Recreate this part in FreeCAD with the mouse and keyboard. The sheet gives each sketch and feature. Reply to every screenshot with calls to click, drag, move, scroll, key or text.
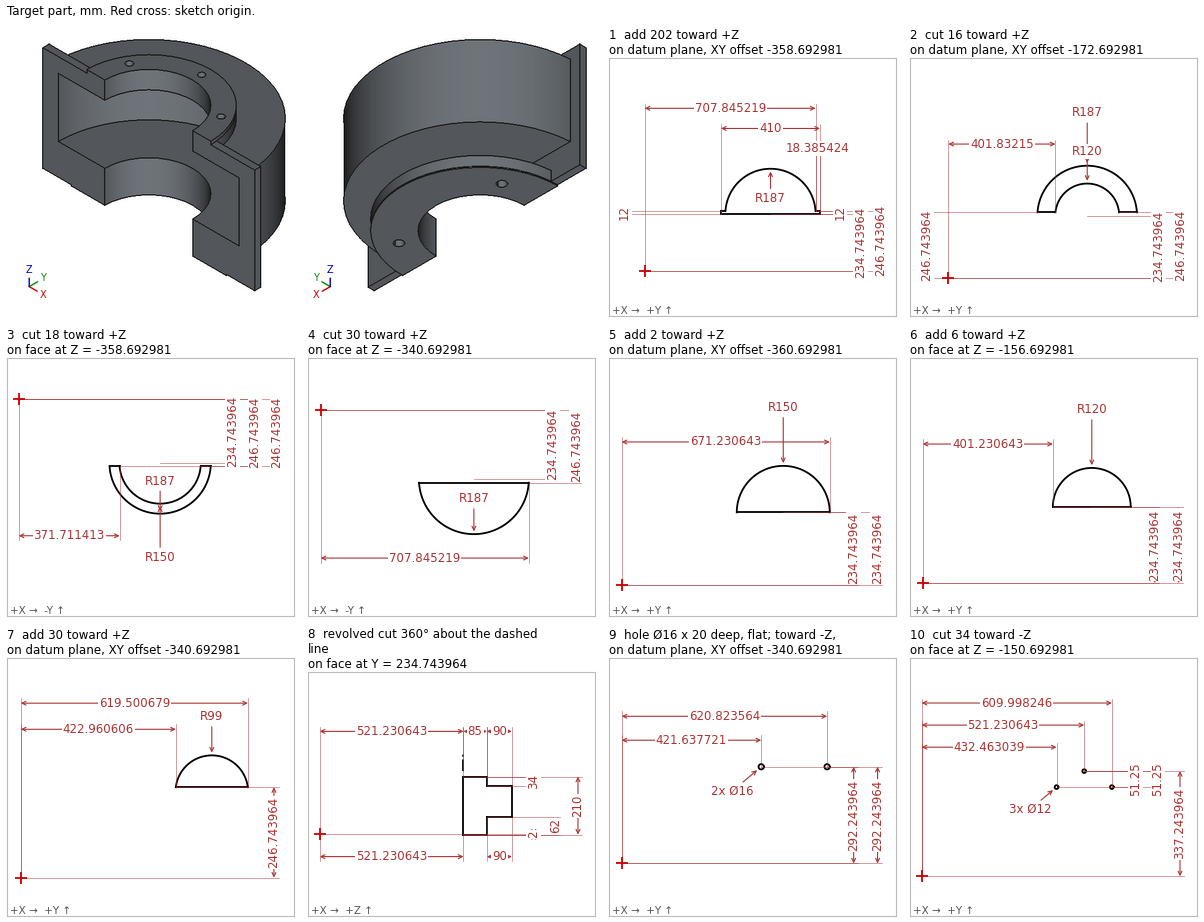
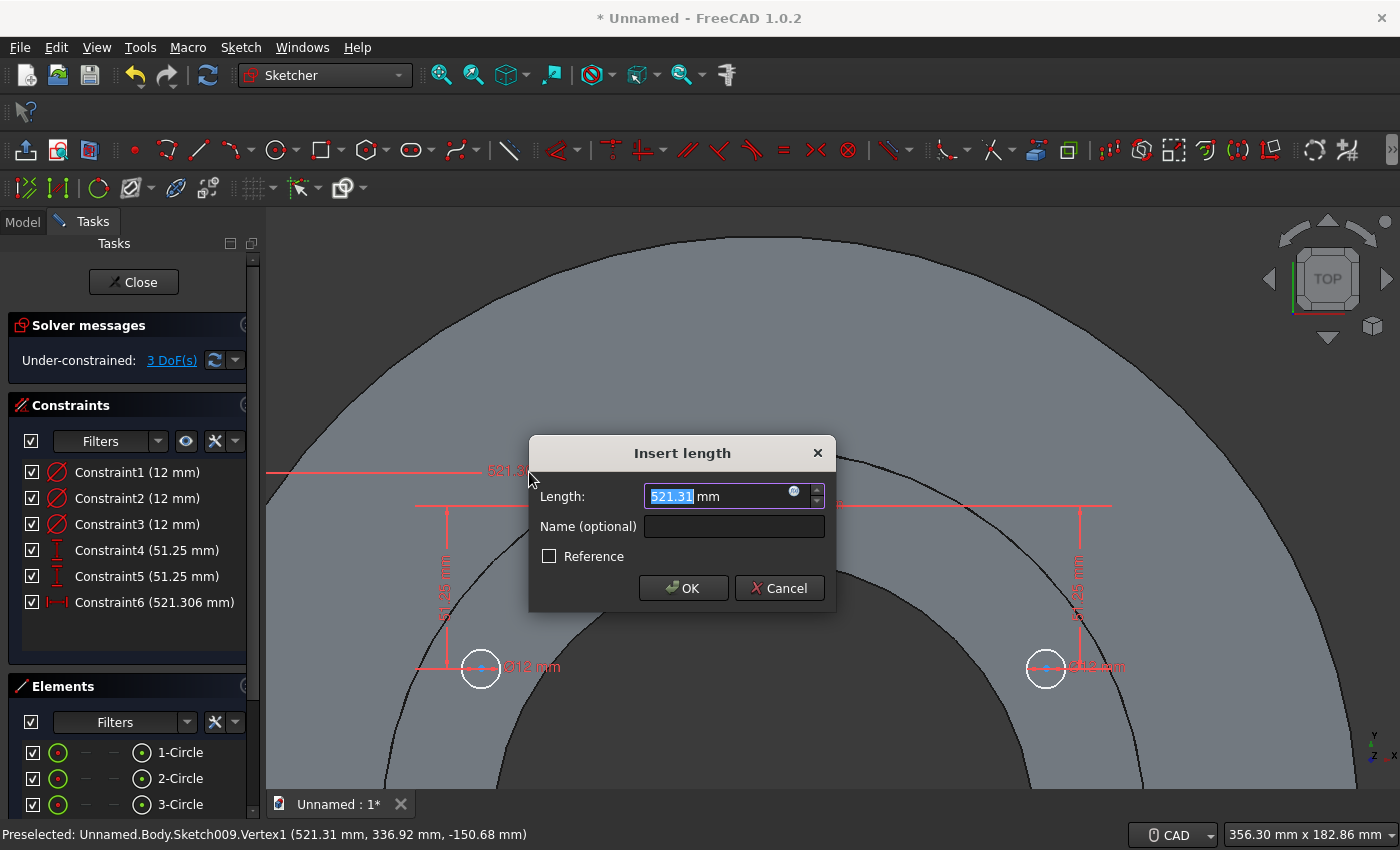
text(521.230643)
key(Return)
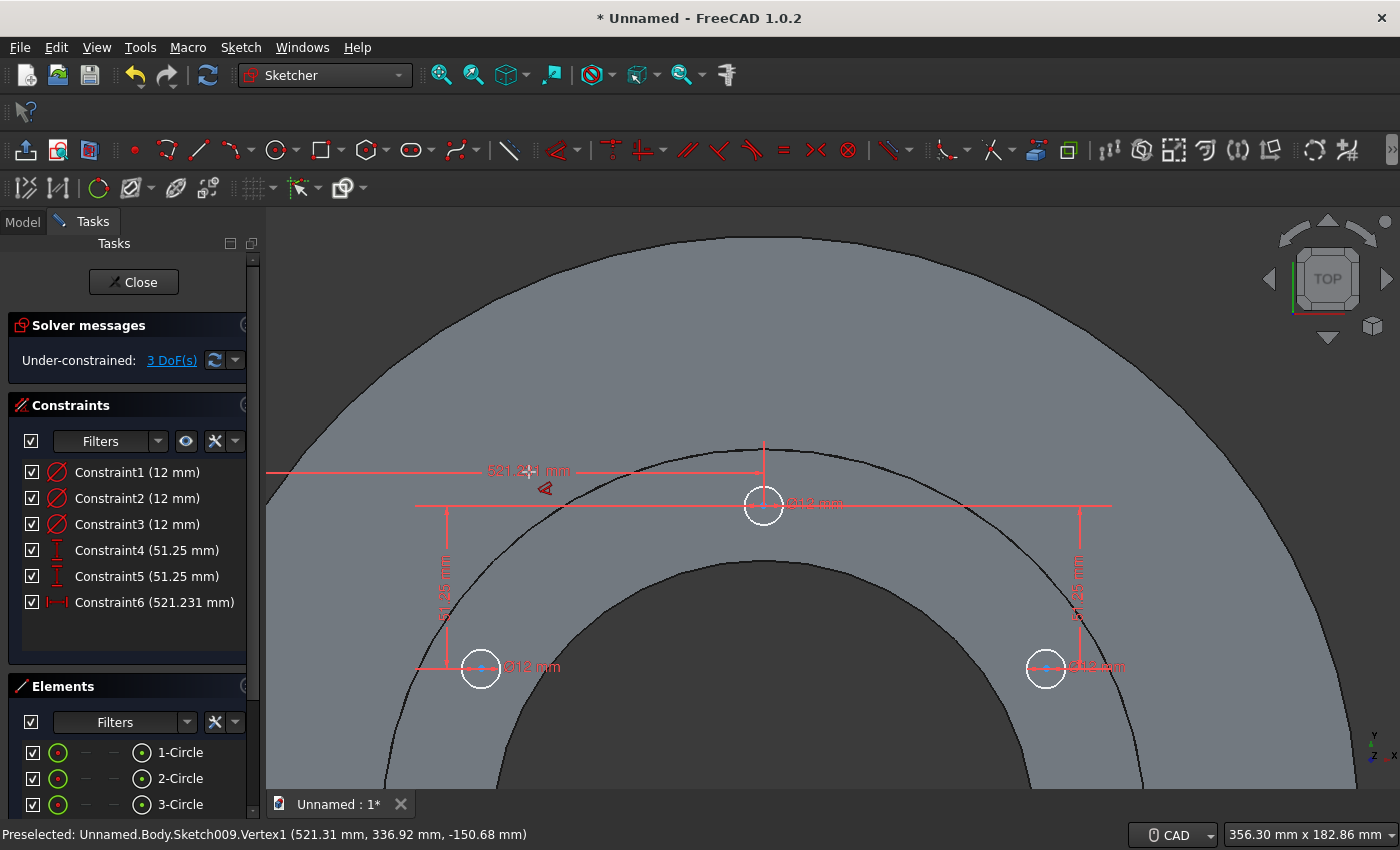
click(764, 506)
click(798, 633)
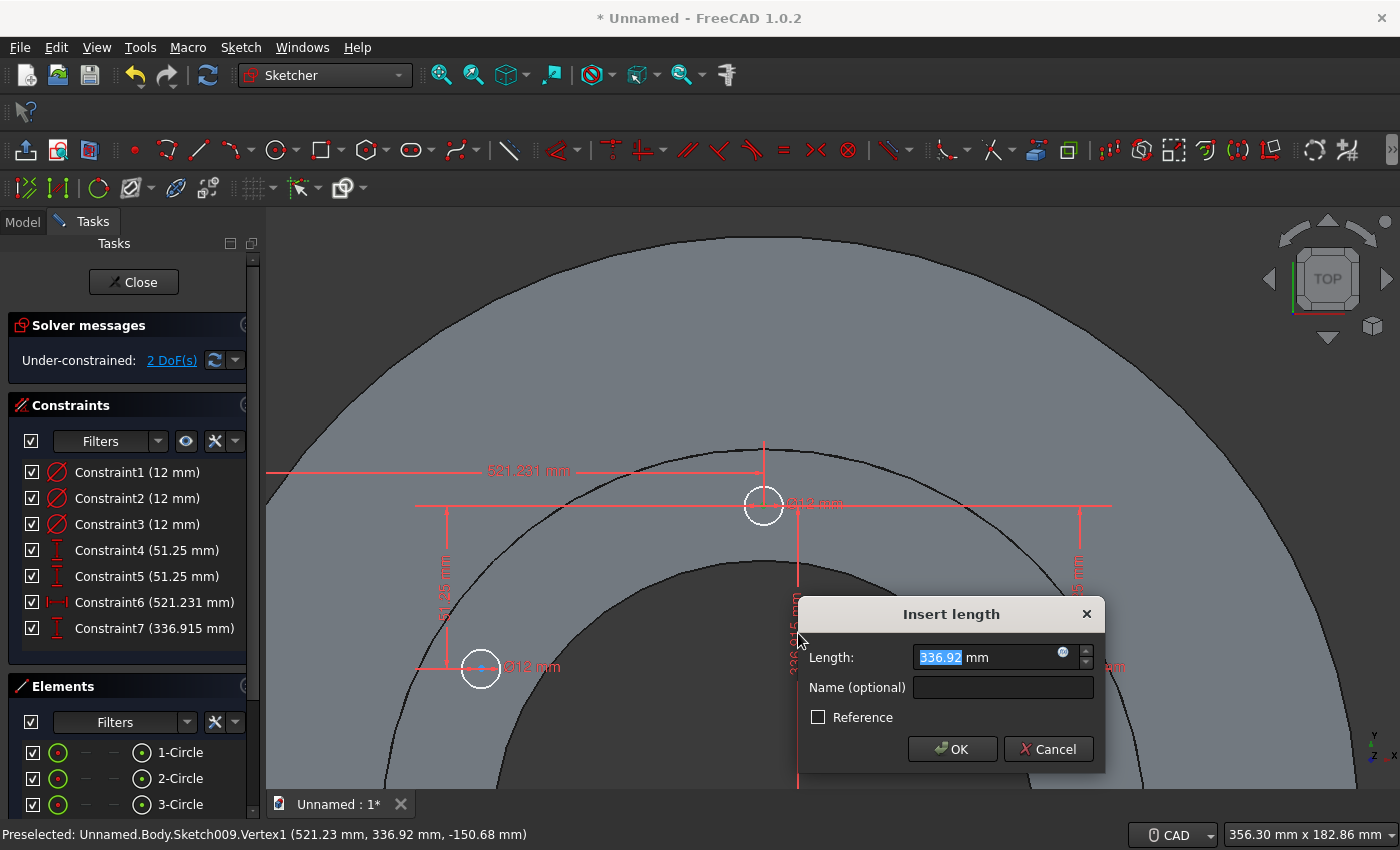
text(337.243964)
key(Return)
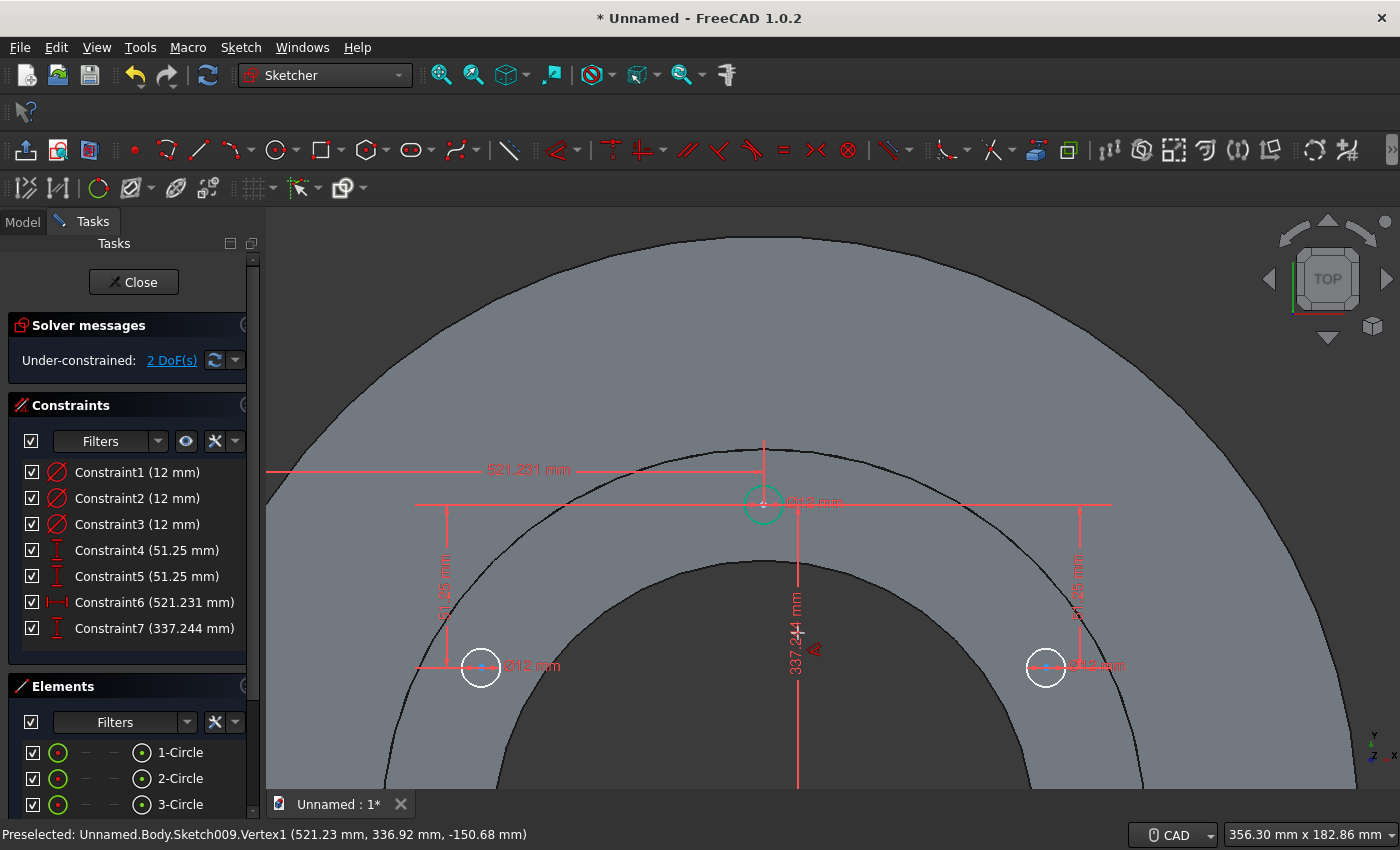
click(481, 668)
click(387, 634)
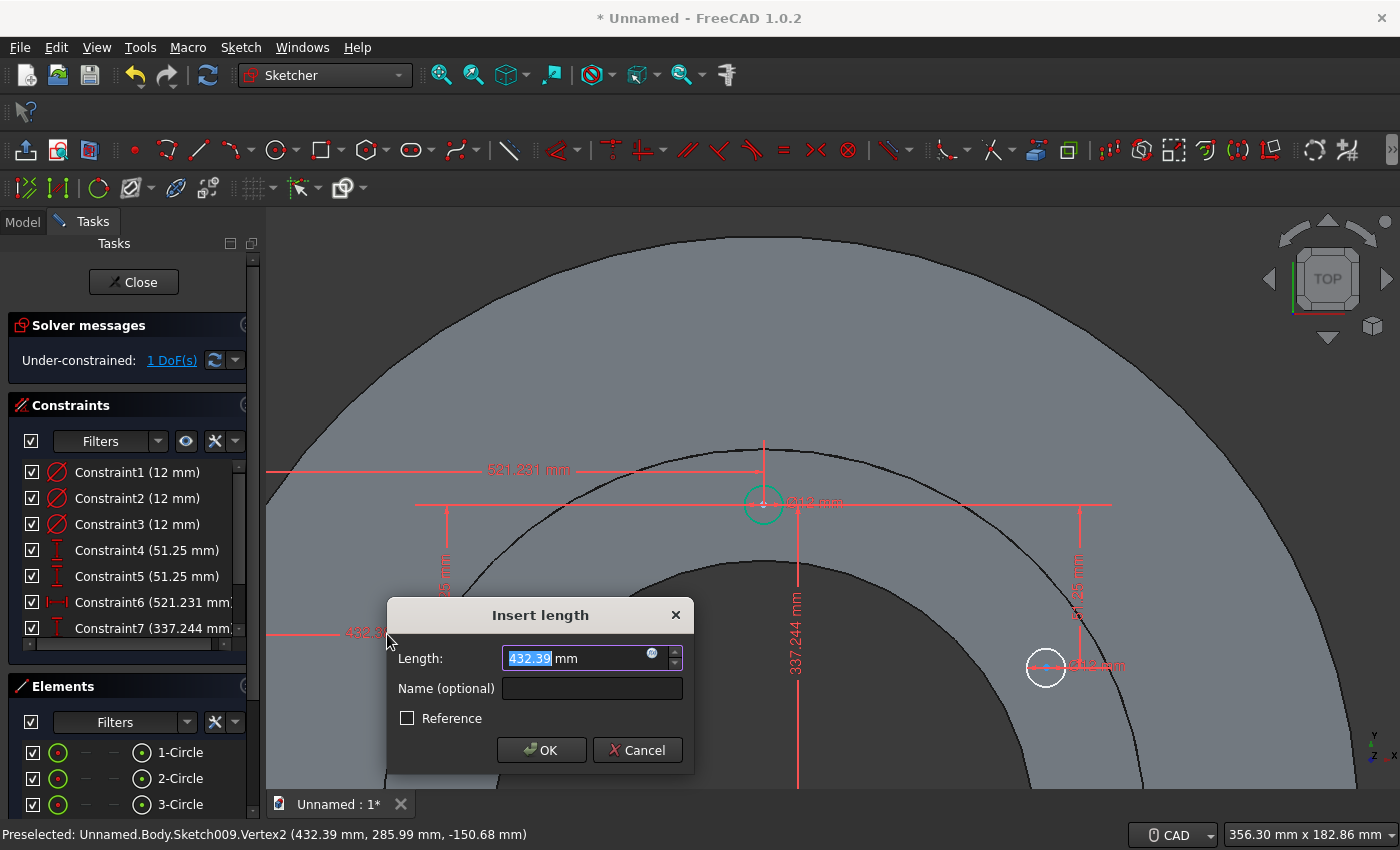
text(432.463039)
key(Return)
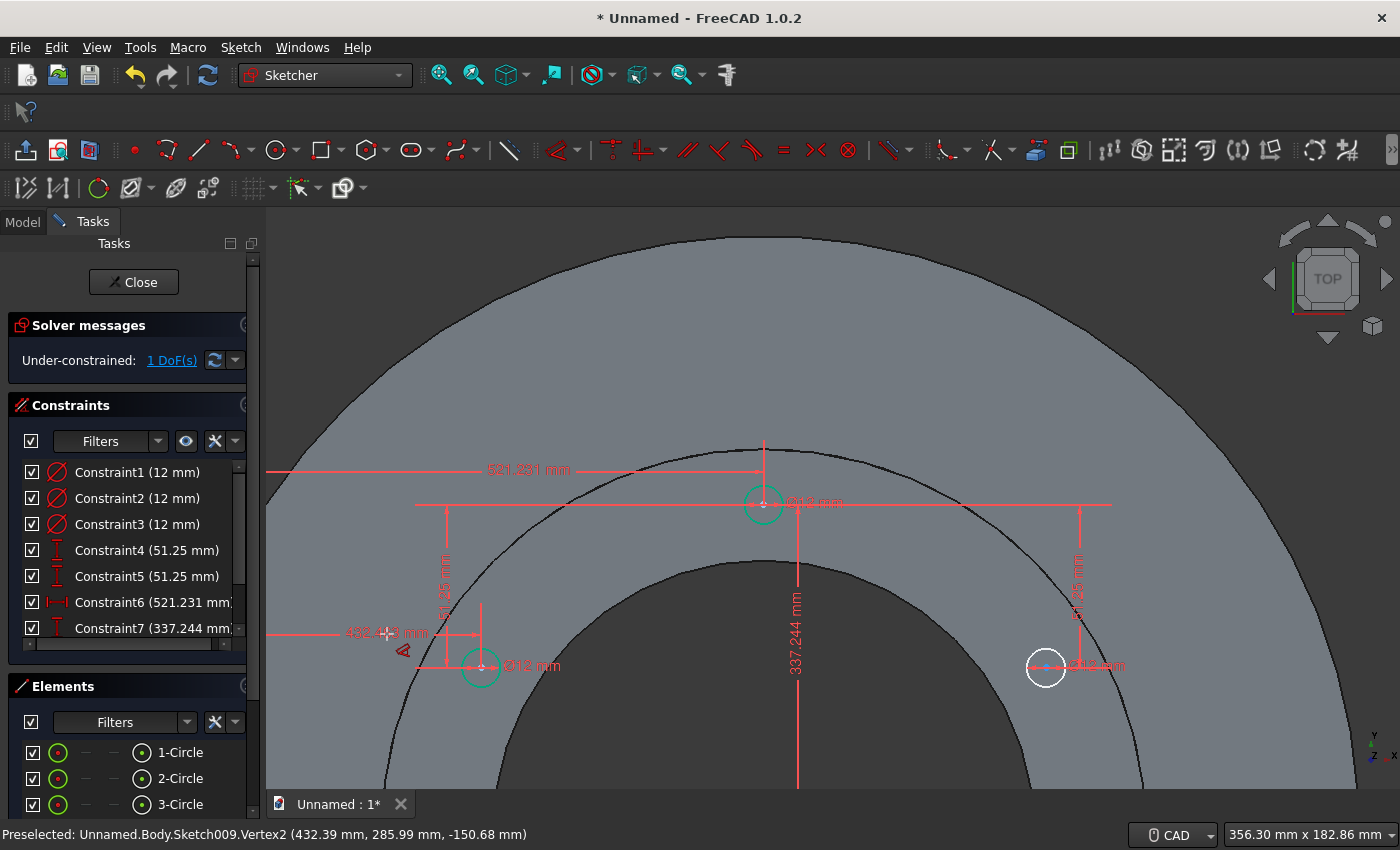
click(1046, 668)
click(670, 634)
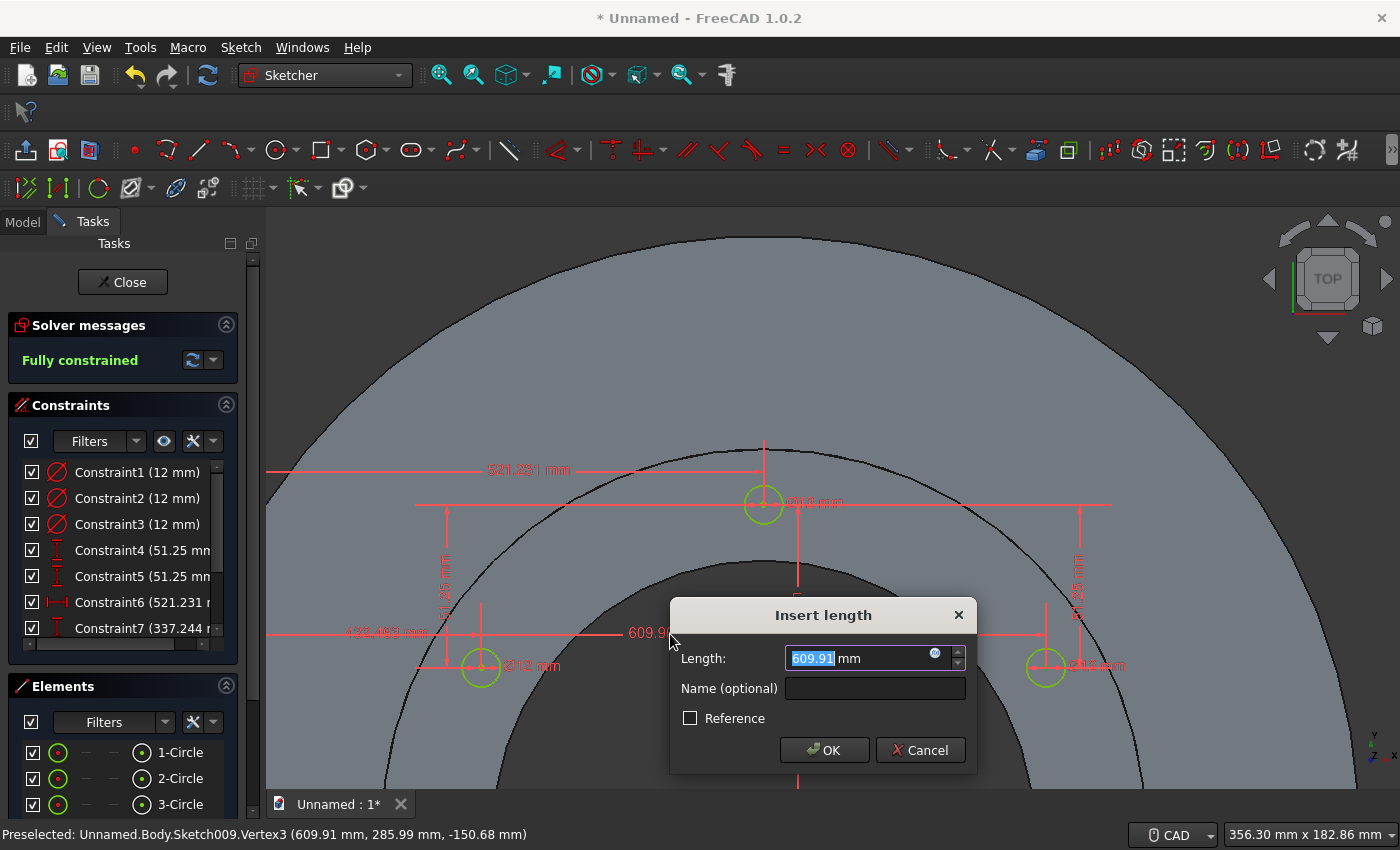
text(609.998246)
key(Return)
key(Escape)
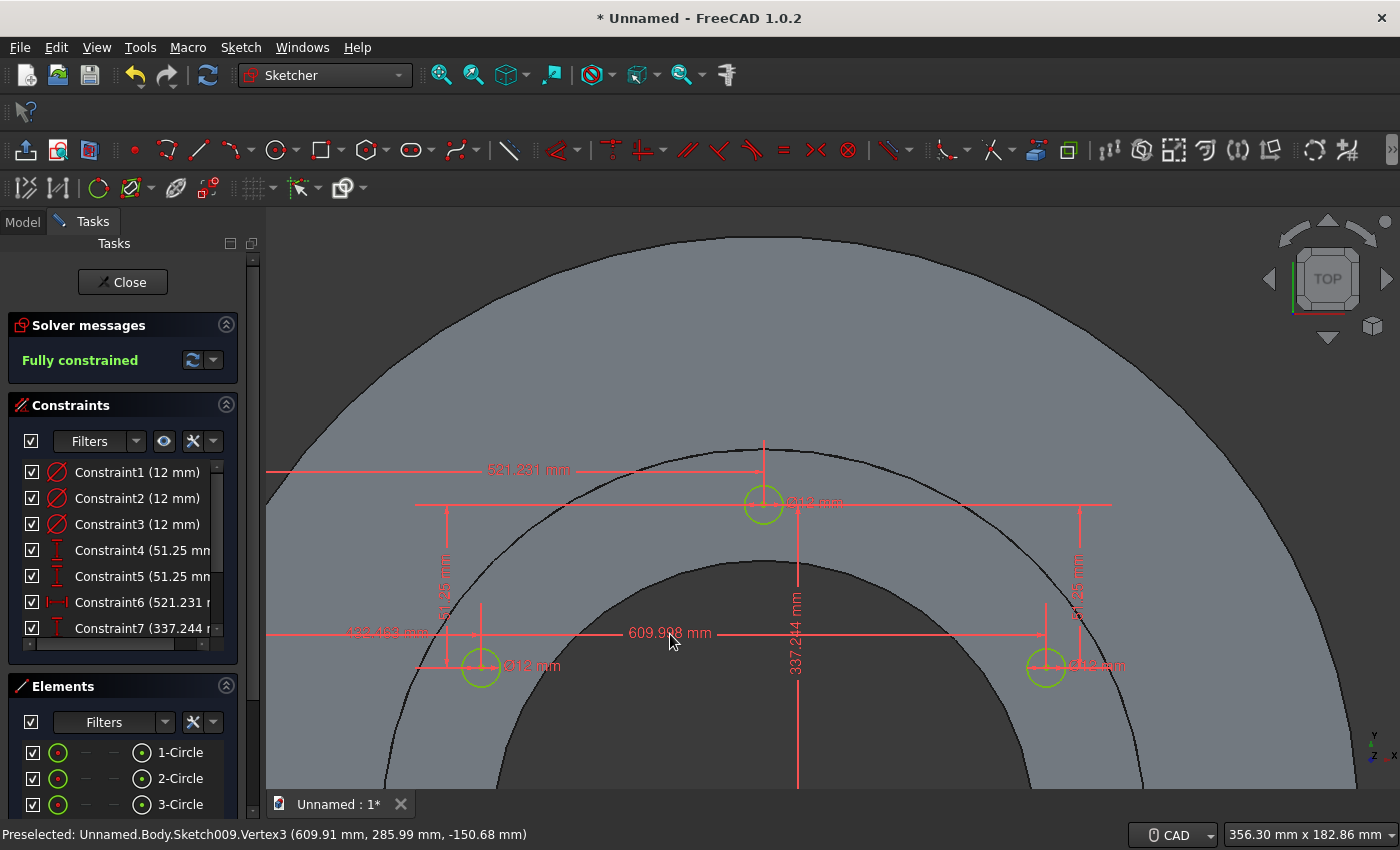
click(123, 282)